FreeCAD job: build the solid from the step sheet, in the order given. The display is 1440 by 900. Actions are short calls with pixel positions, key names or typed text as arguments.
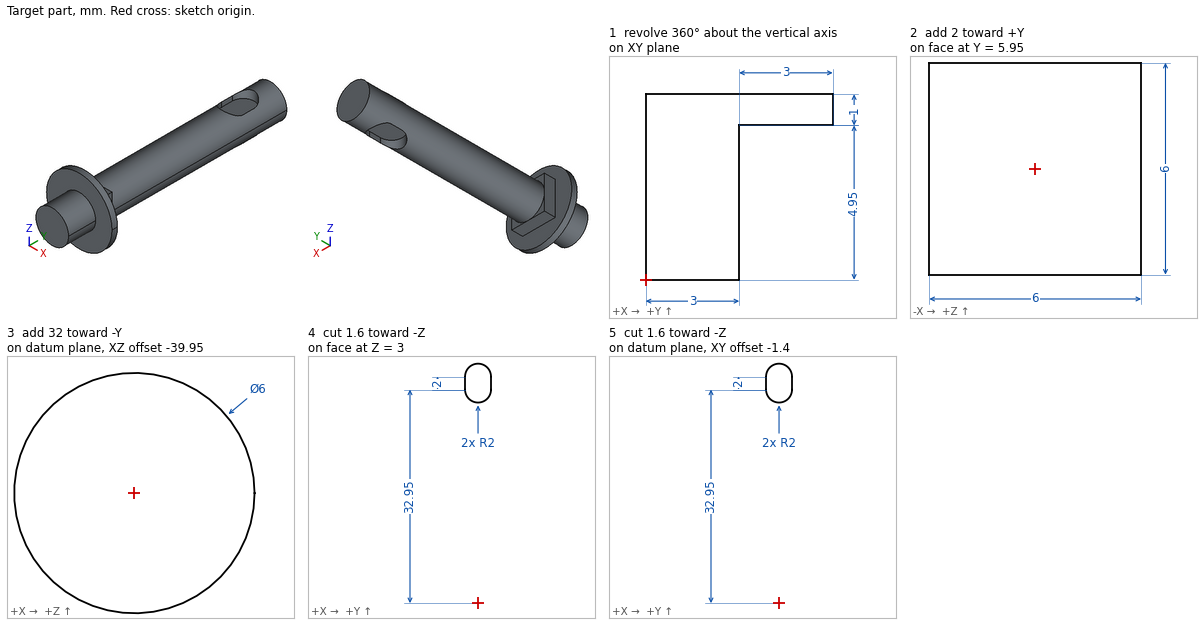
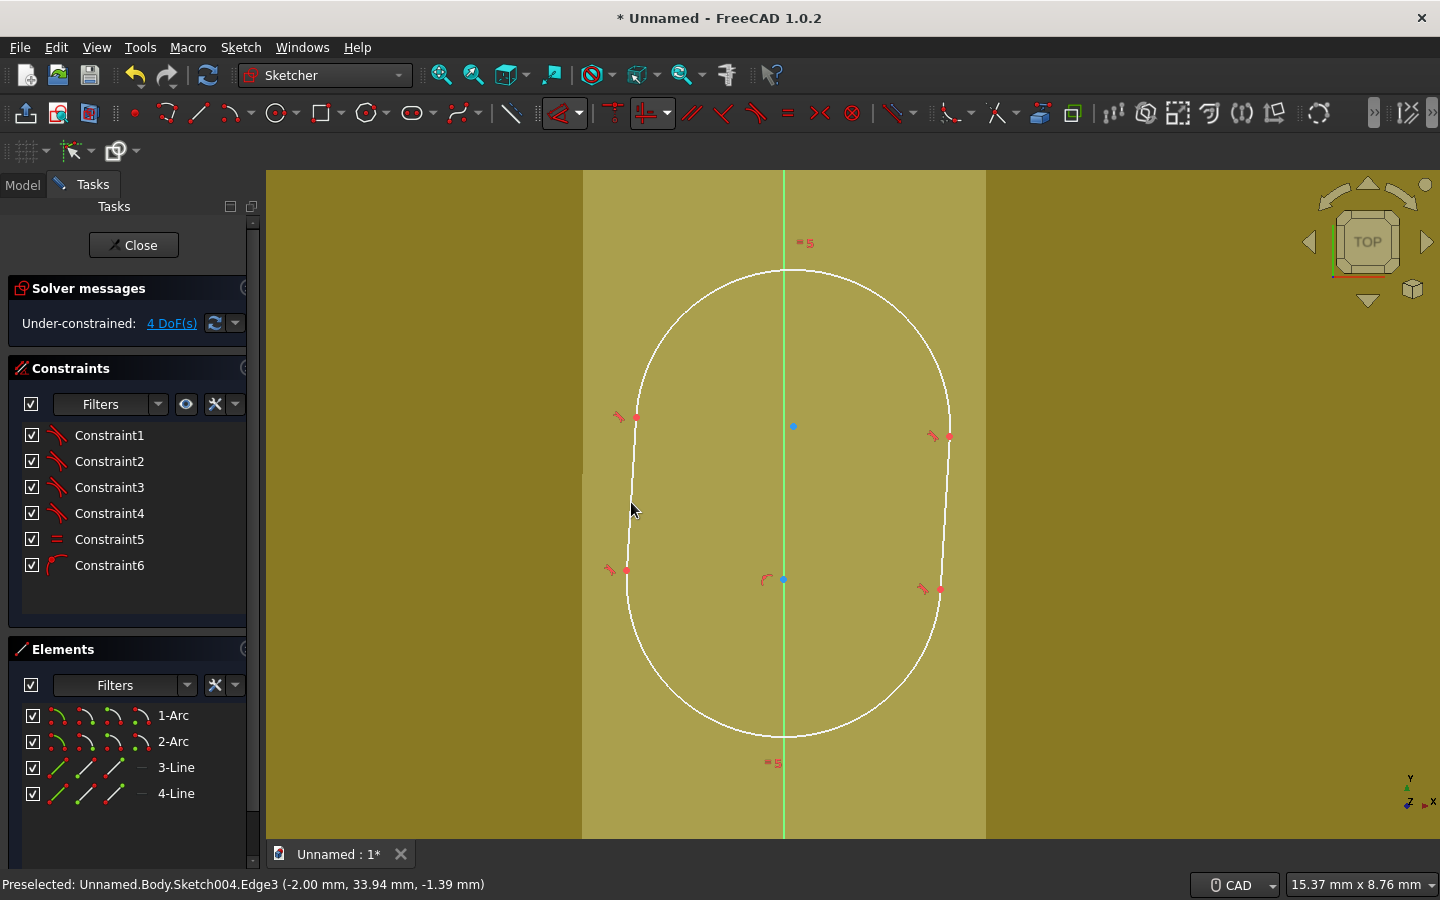
click(630, 525)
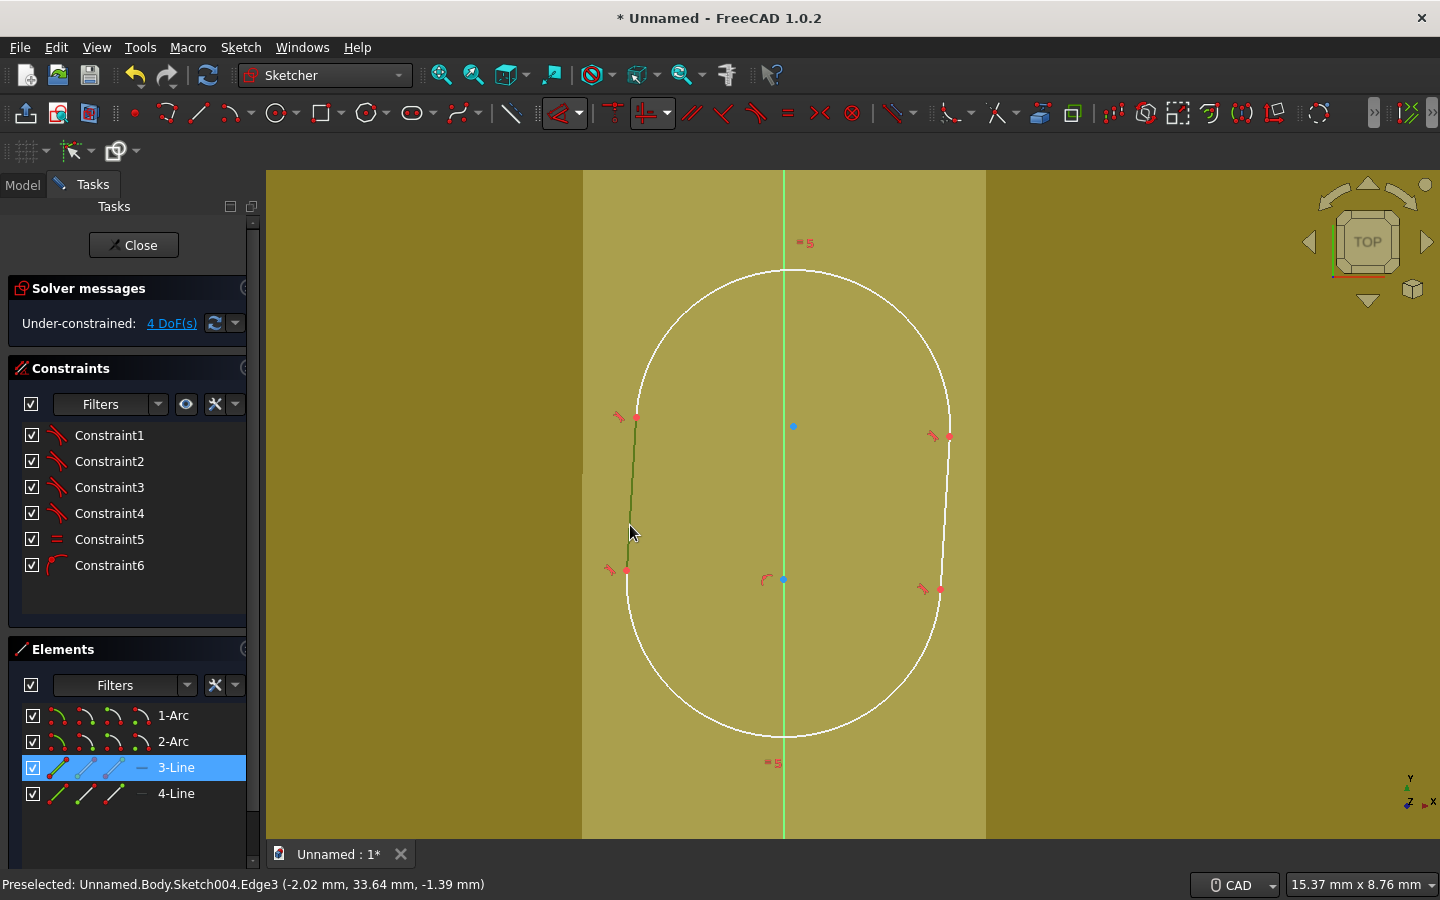
key(v)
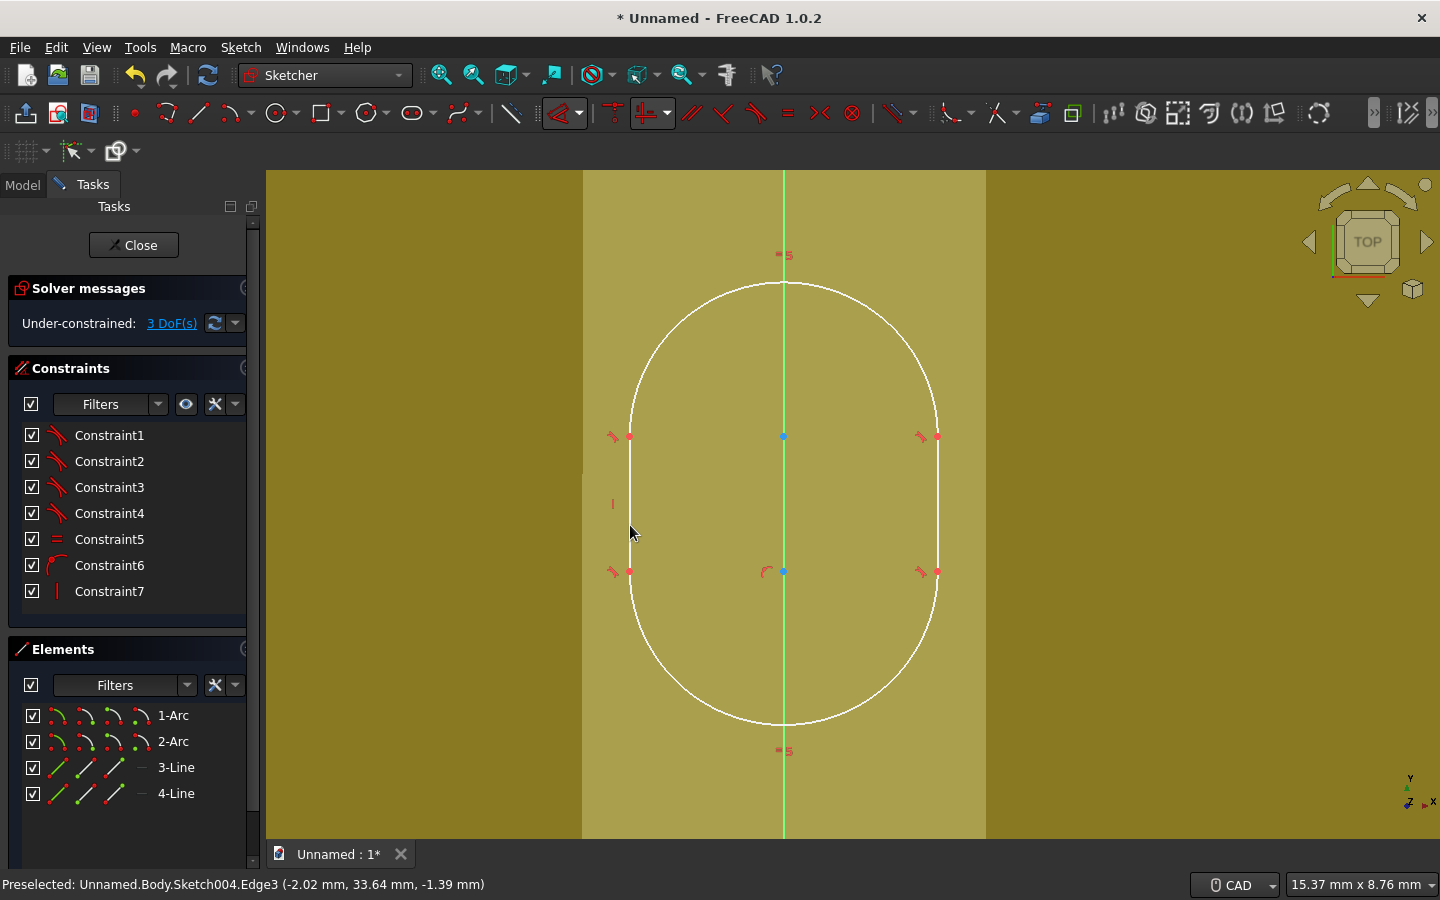
click(693, 696)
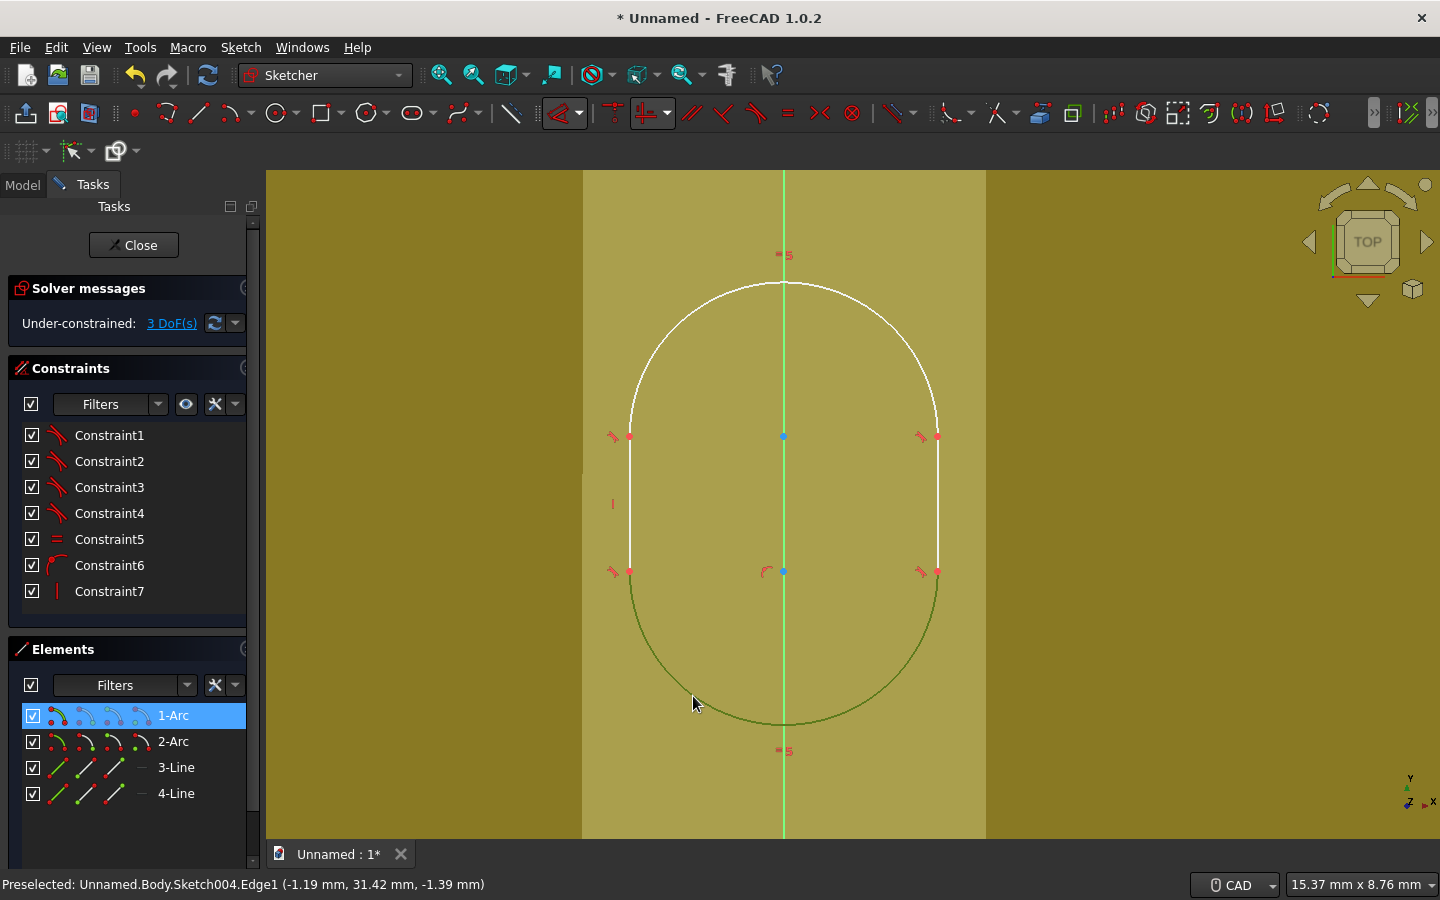
key(k)
key(r)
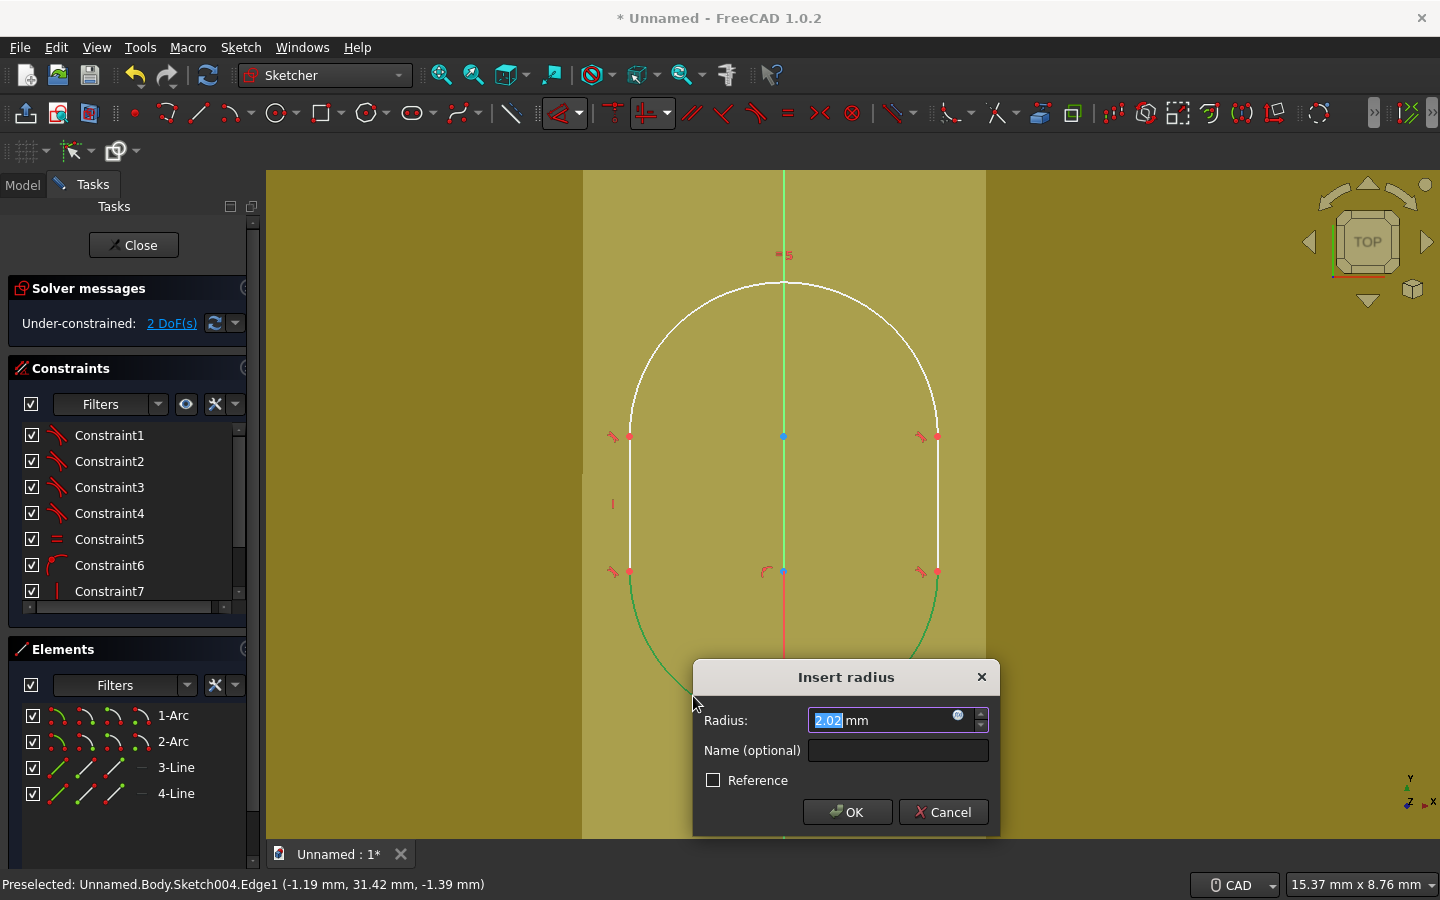
text(2)
key(Return)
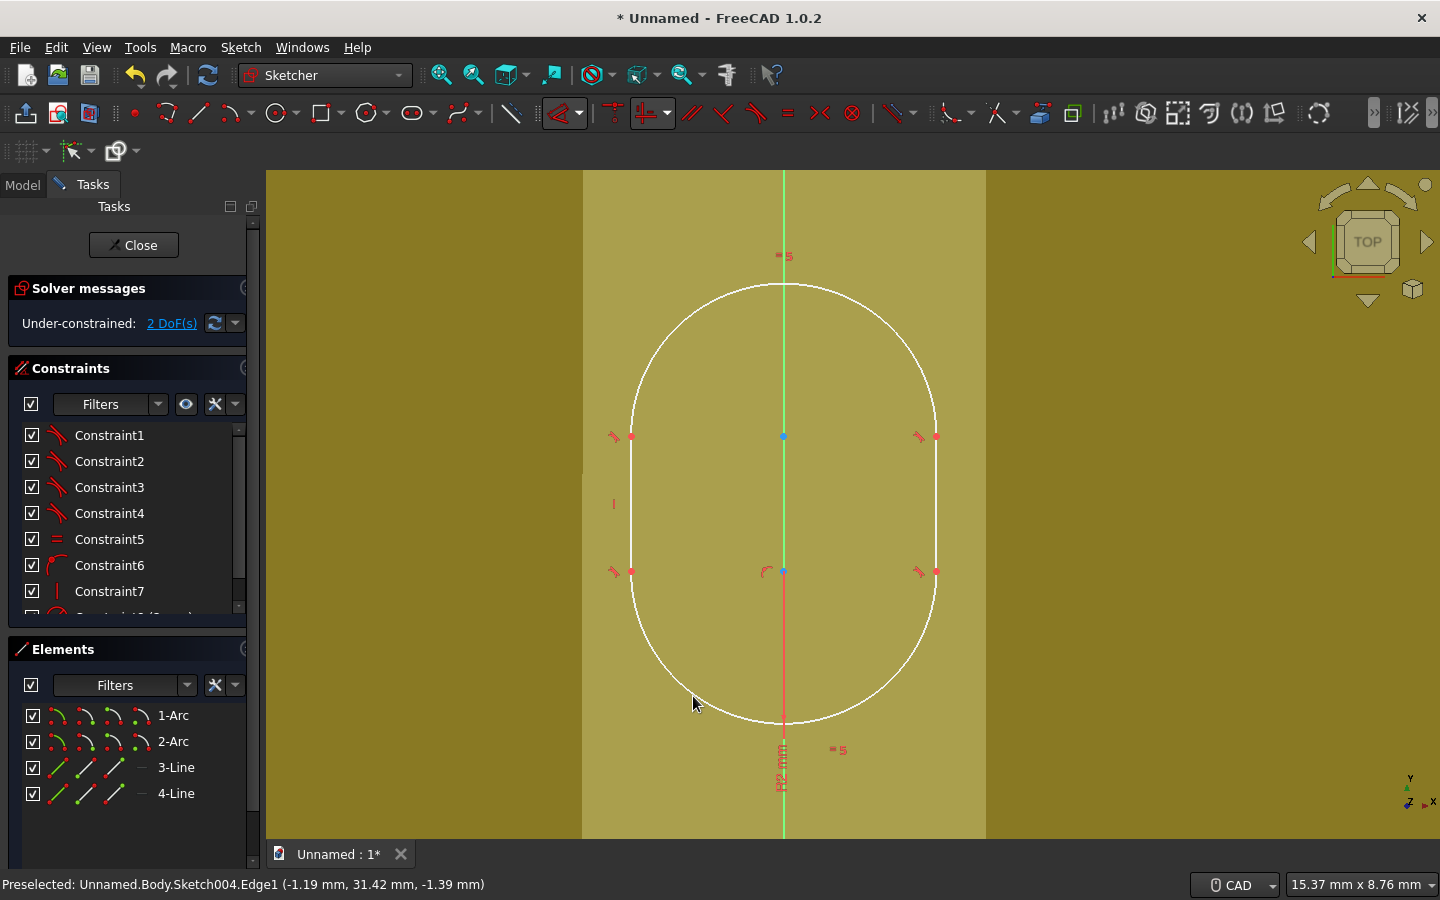
click(631, 531)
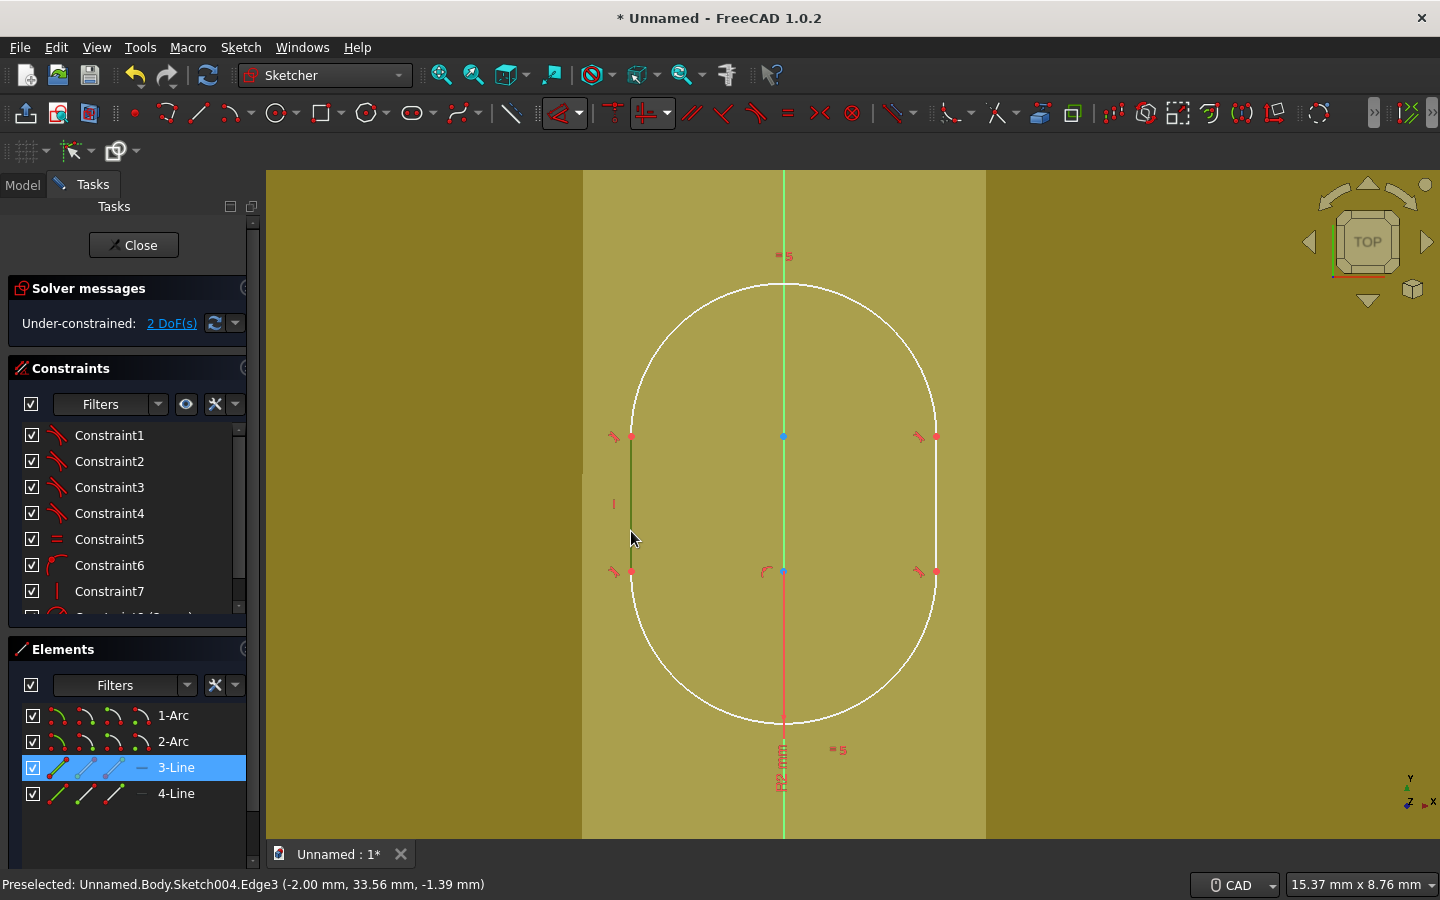
key(i)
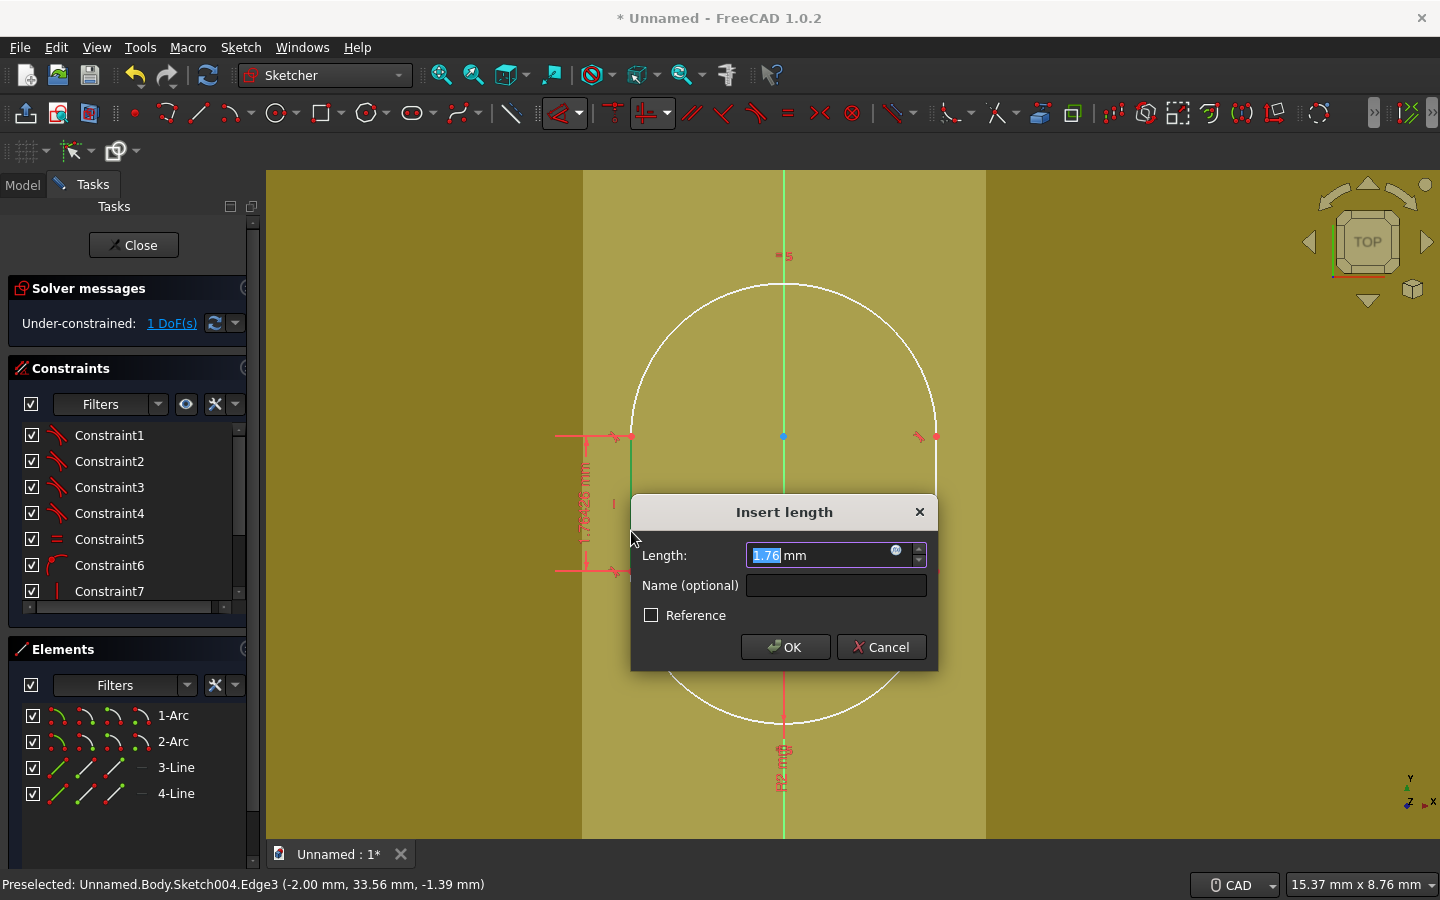
text(2)
key(Return)